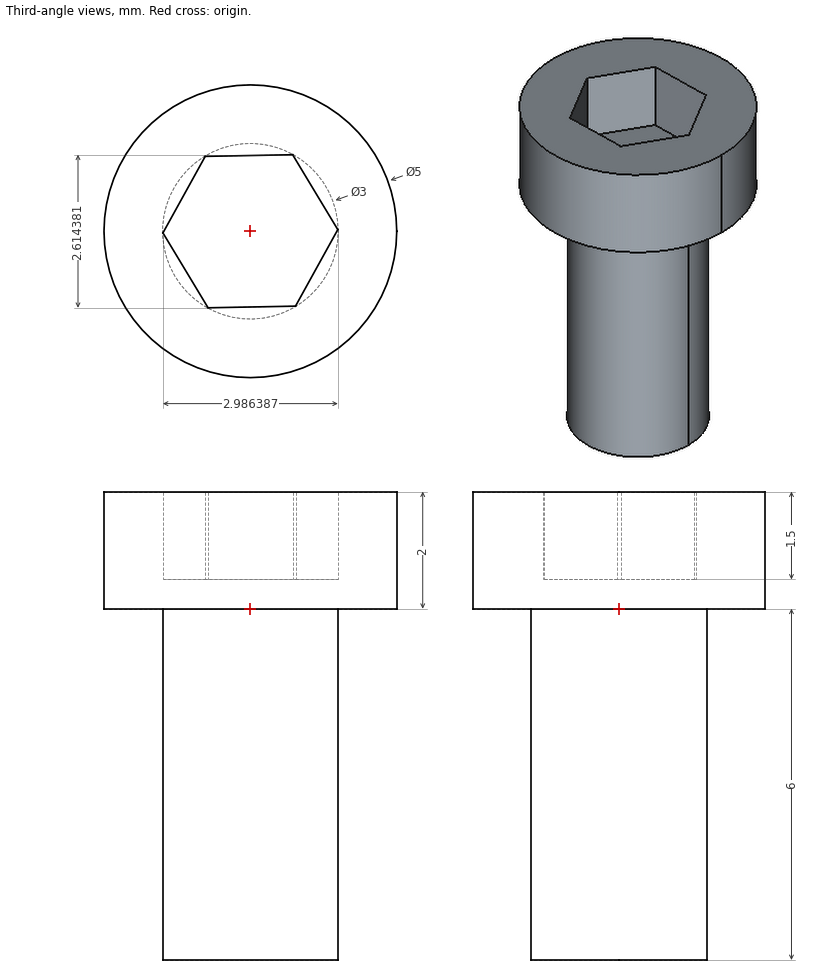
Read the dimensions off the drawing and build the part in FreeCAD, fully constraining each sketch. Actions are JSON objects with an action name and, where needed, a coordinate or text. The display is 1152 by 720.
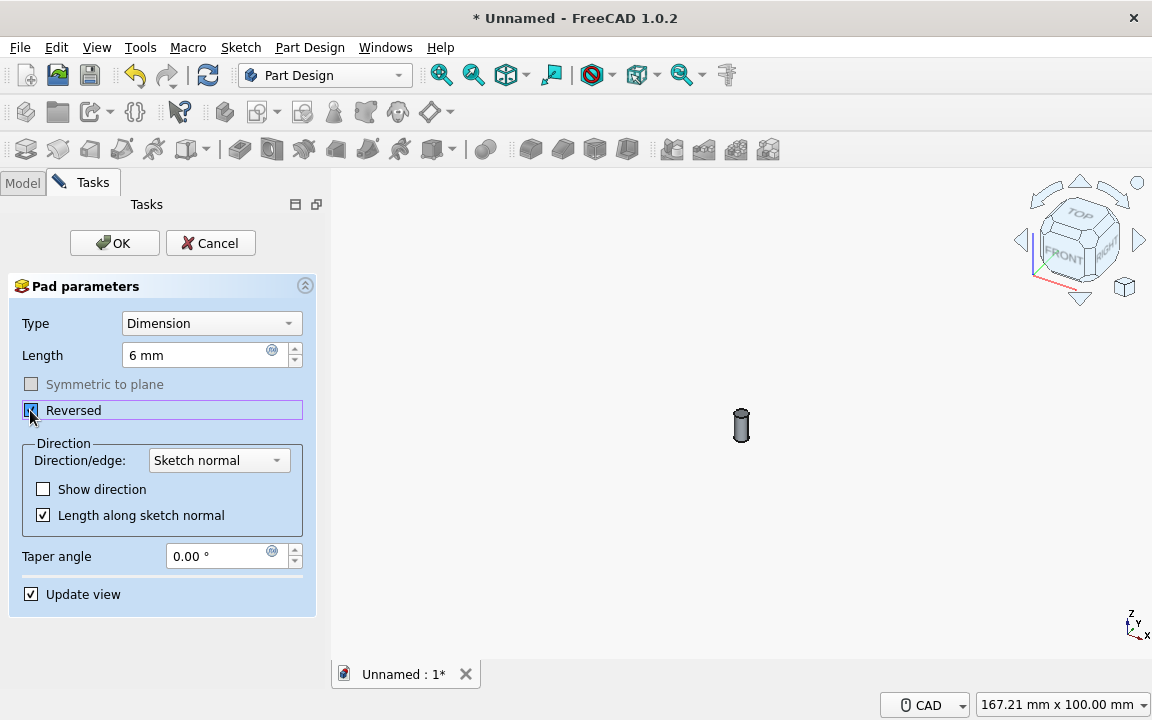
{"action": "left_click", "coordinate": [115, 243]}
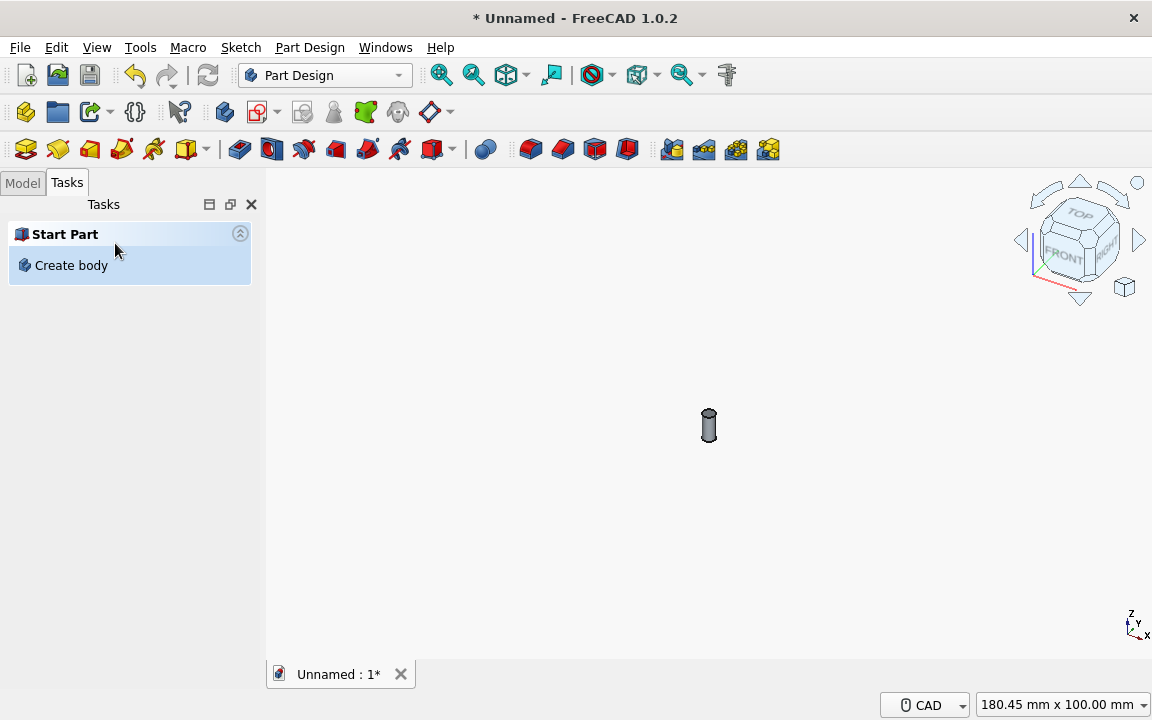
{"action": "left_click", "coordinate": [442, 76]}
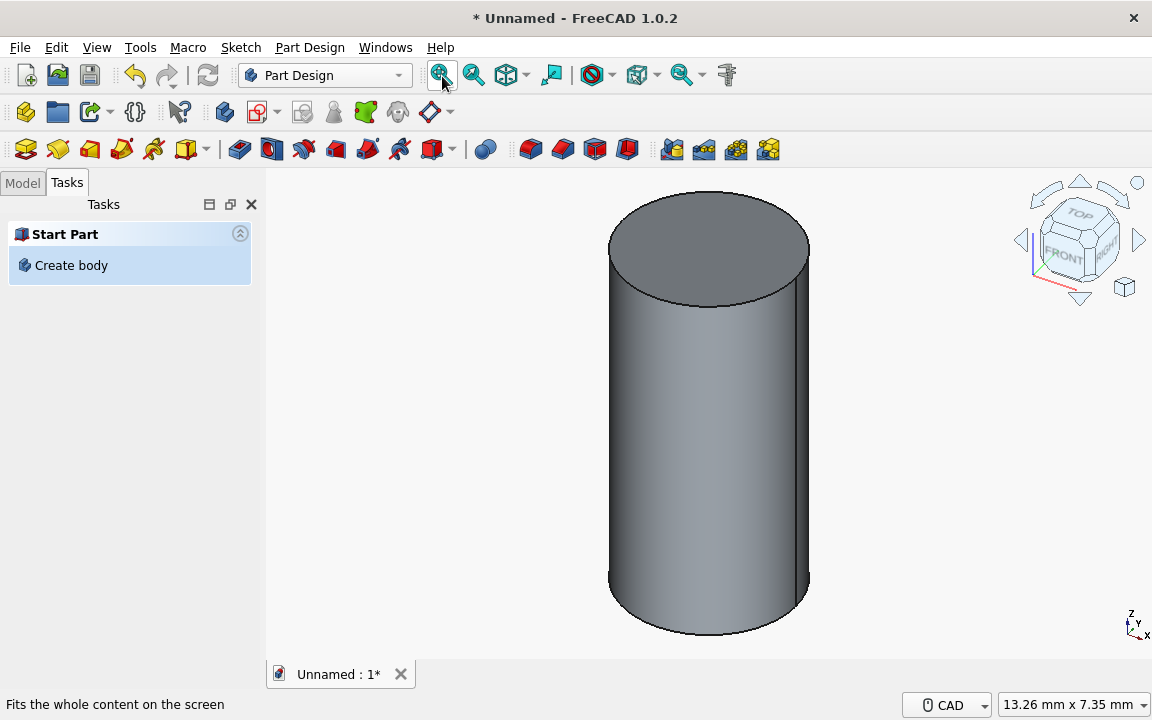
{"action": "left_click", "coordinate": [709, 248]}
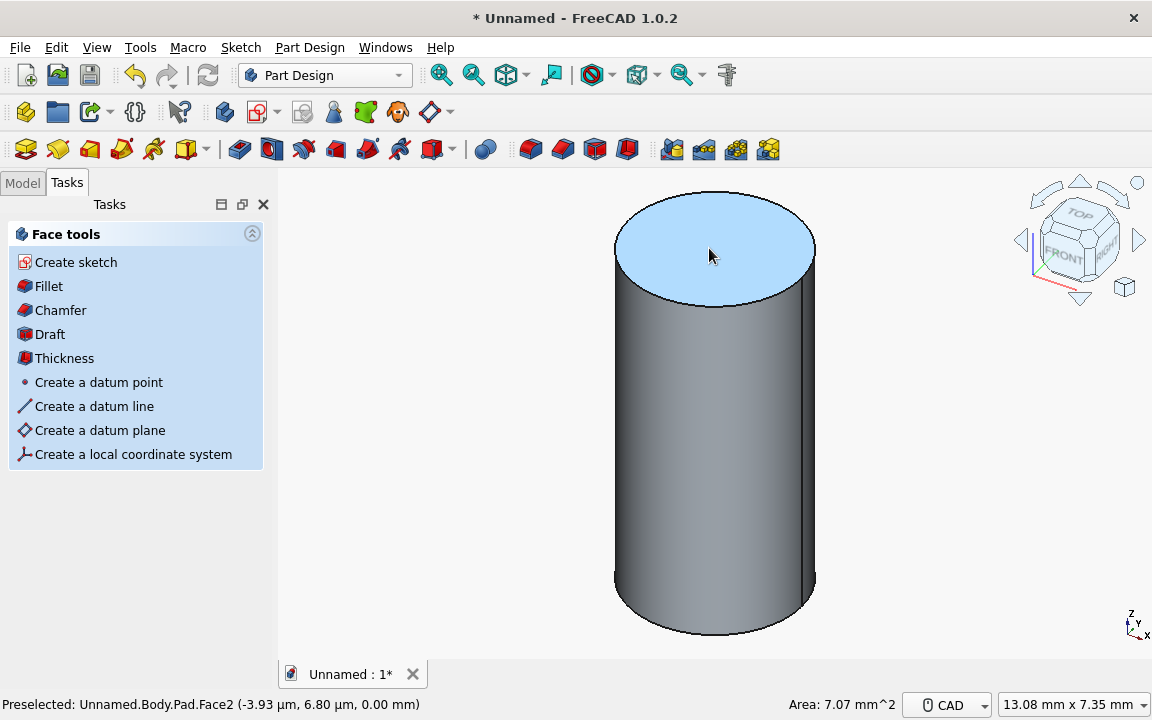
{"action": "left_click", "coordinate": [258, 112]}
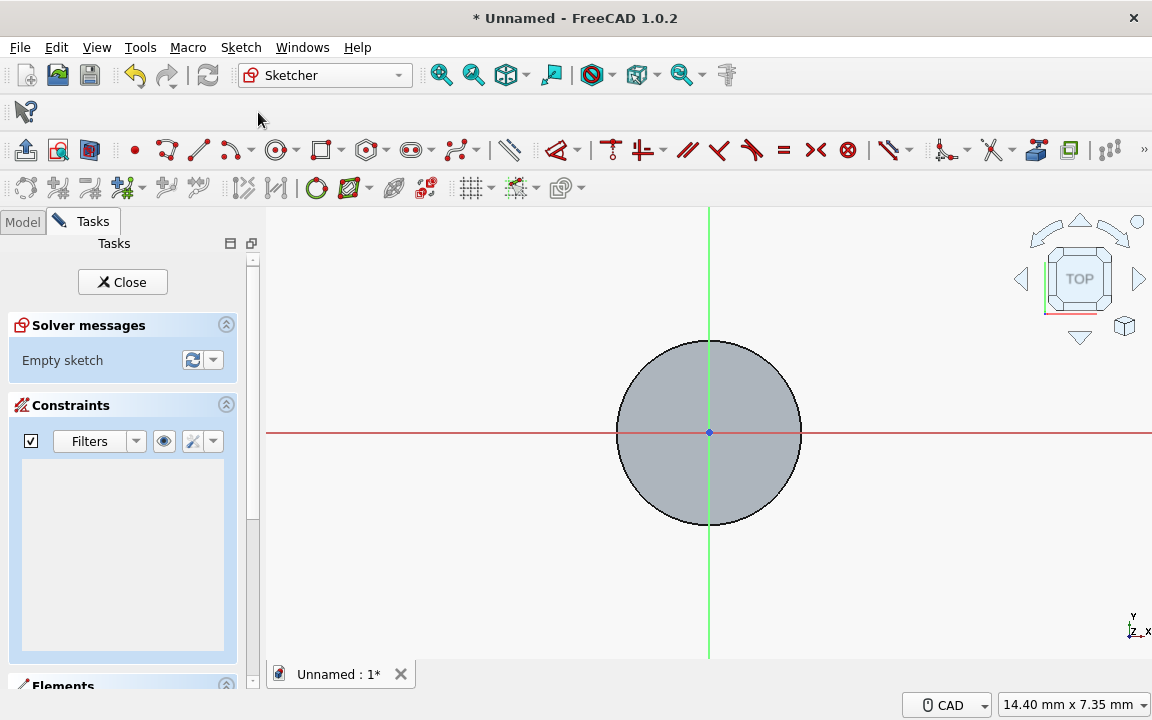
{"action": "left_click", "coordinate": [276, 150]}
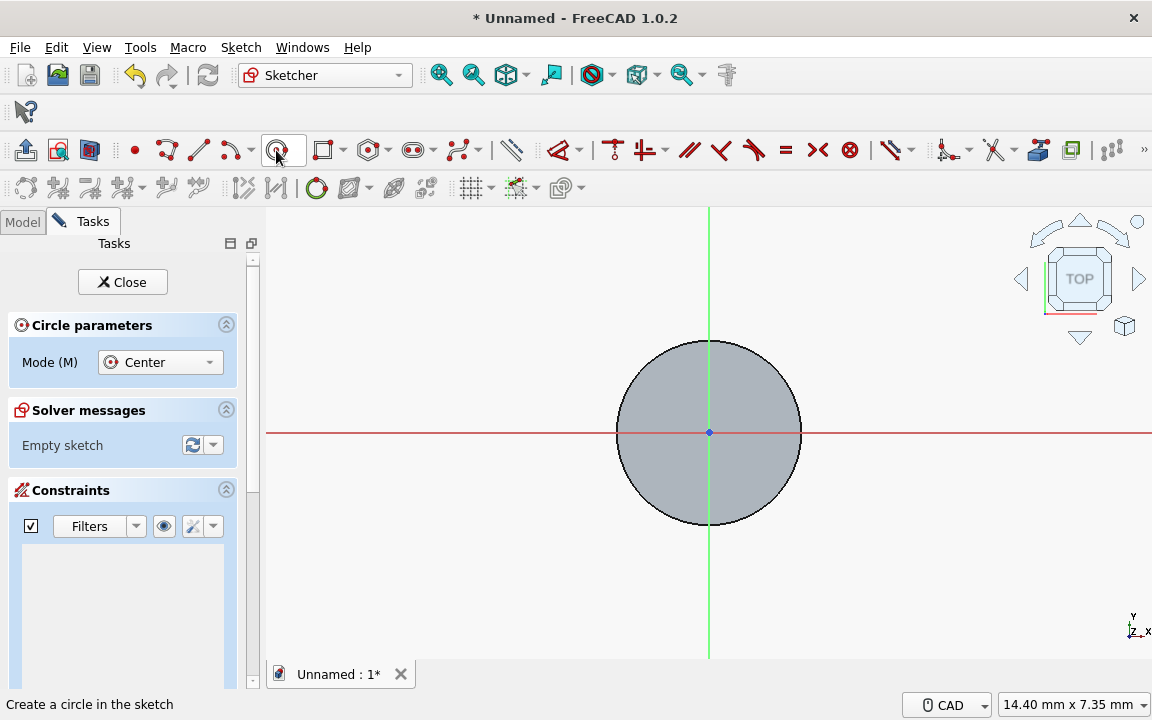
{"action": "left_click", "coordinate": [709, 433]}
{"action": "mouse_move", "coordinate": [818, 324]}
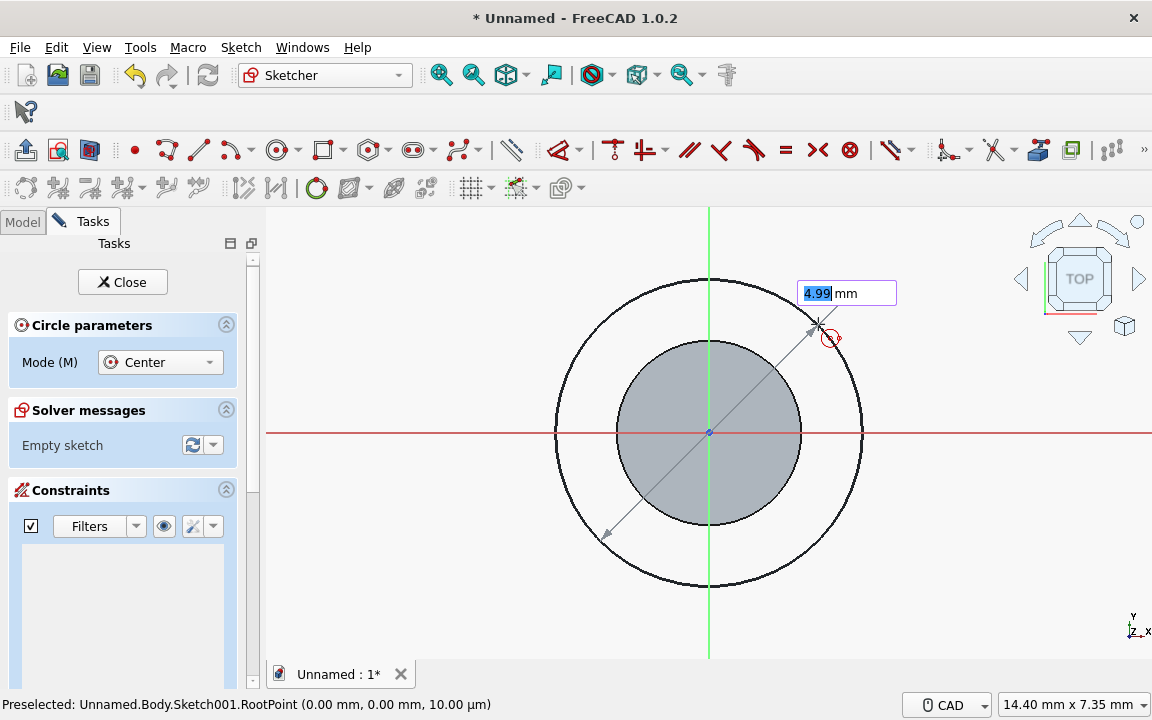
{"action": "type", "text": "5"}
{"action": "key", "text": "Return"}
{"action": "key", "text": "Escape"}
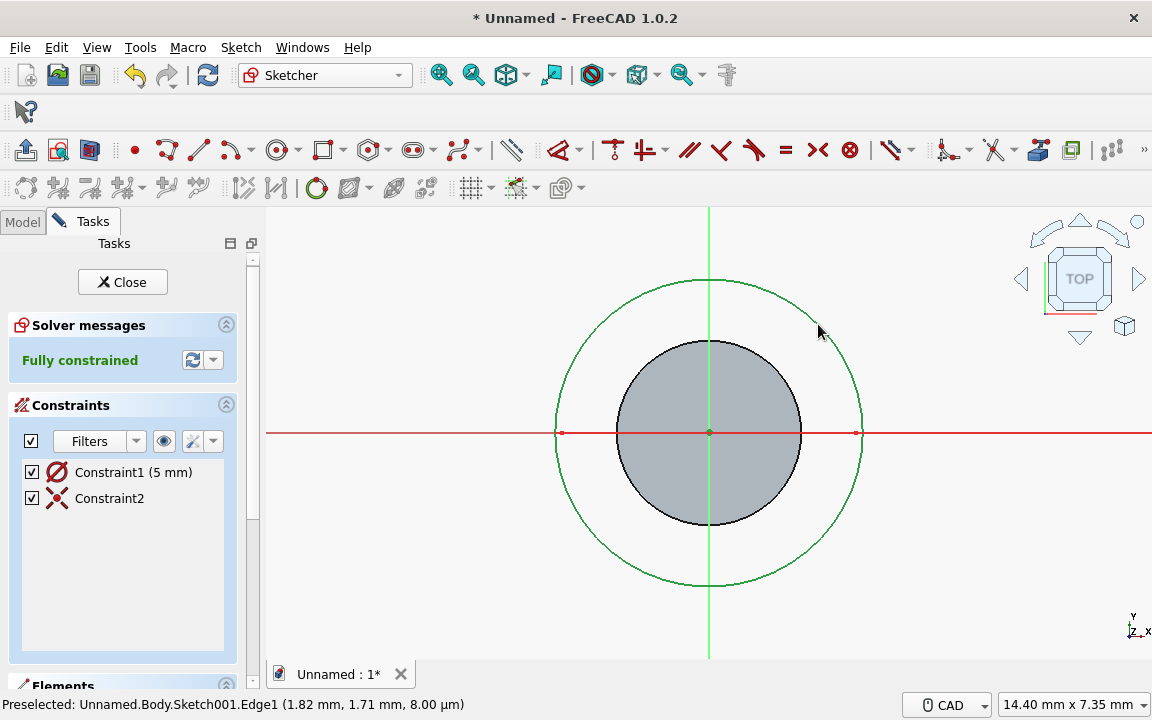
{"action": "left_click", "coordinate": [123, 282]}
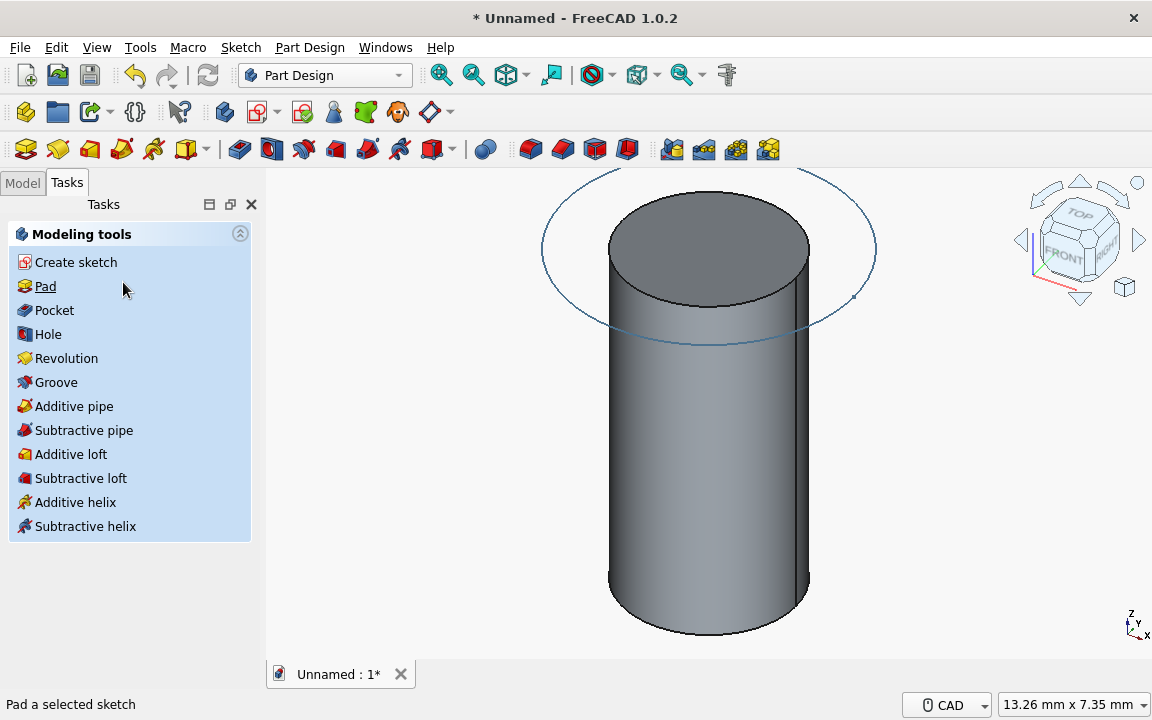
{"action": "left_click", "coordinate": [26, 150]}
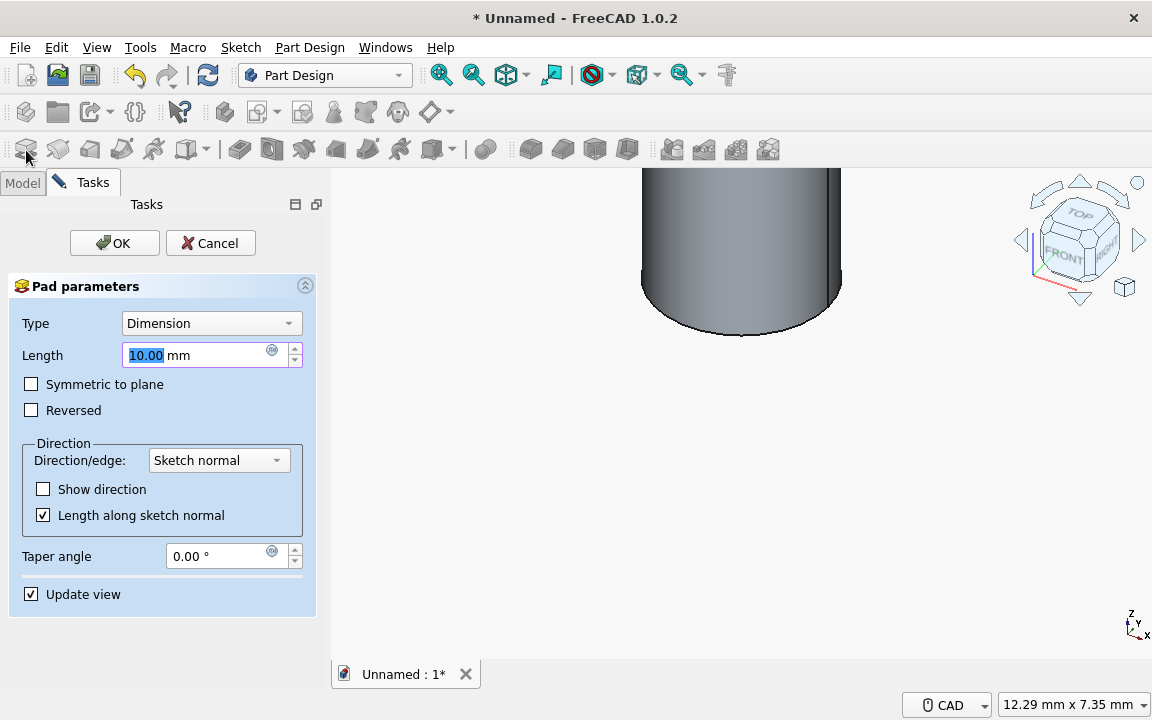
{"action": "type", "text": "2"}
{"action": "key", "text": "Tab"}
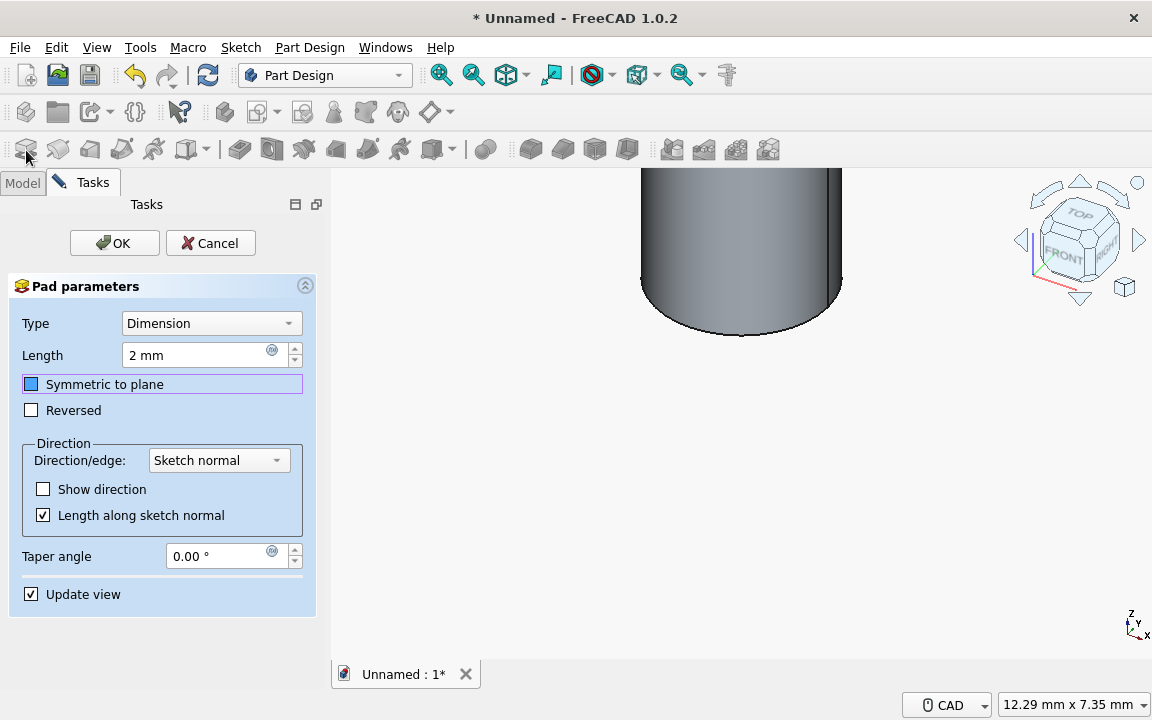
{"action": "left_click", "coordinate": [115, 243]}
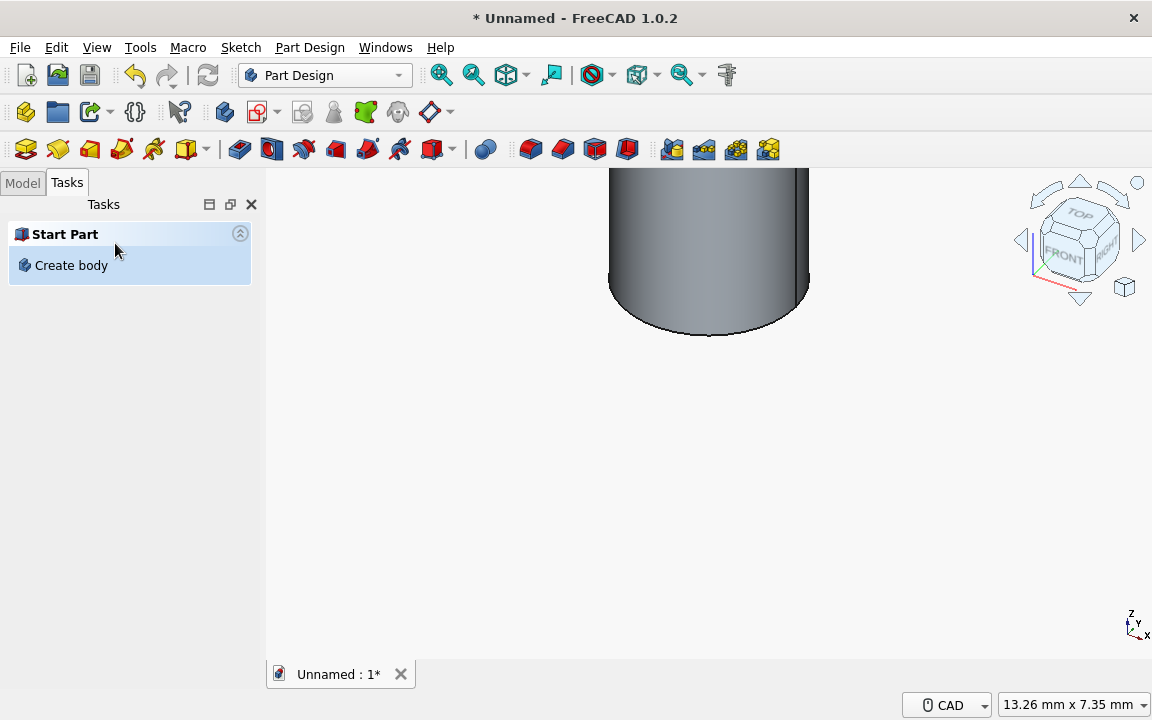
{"action": "left_click", "coordinate": [442, 76]}